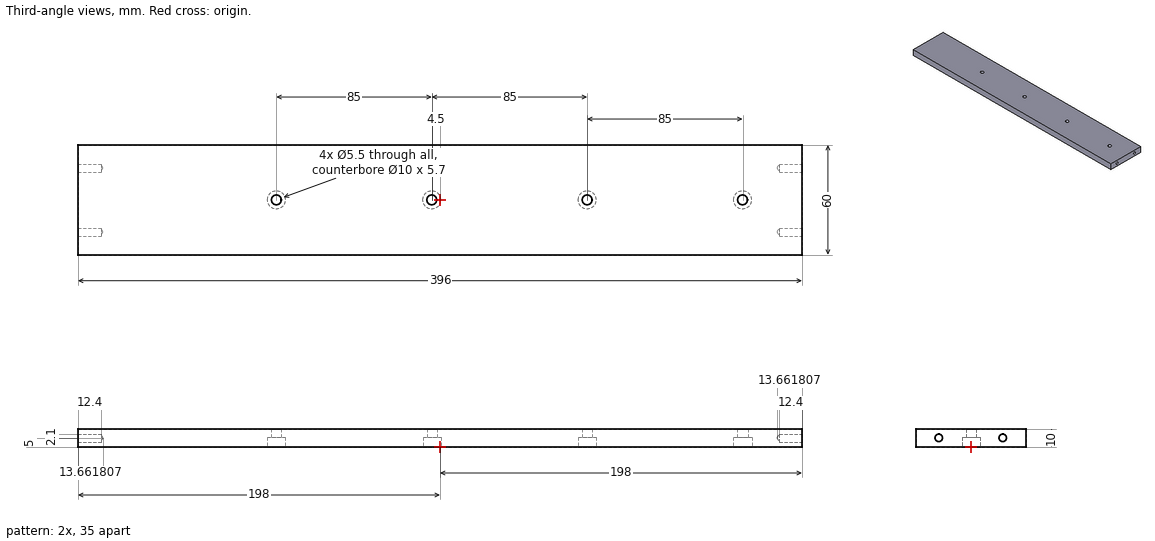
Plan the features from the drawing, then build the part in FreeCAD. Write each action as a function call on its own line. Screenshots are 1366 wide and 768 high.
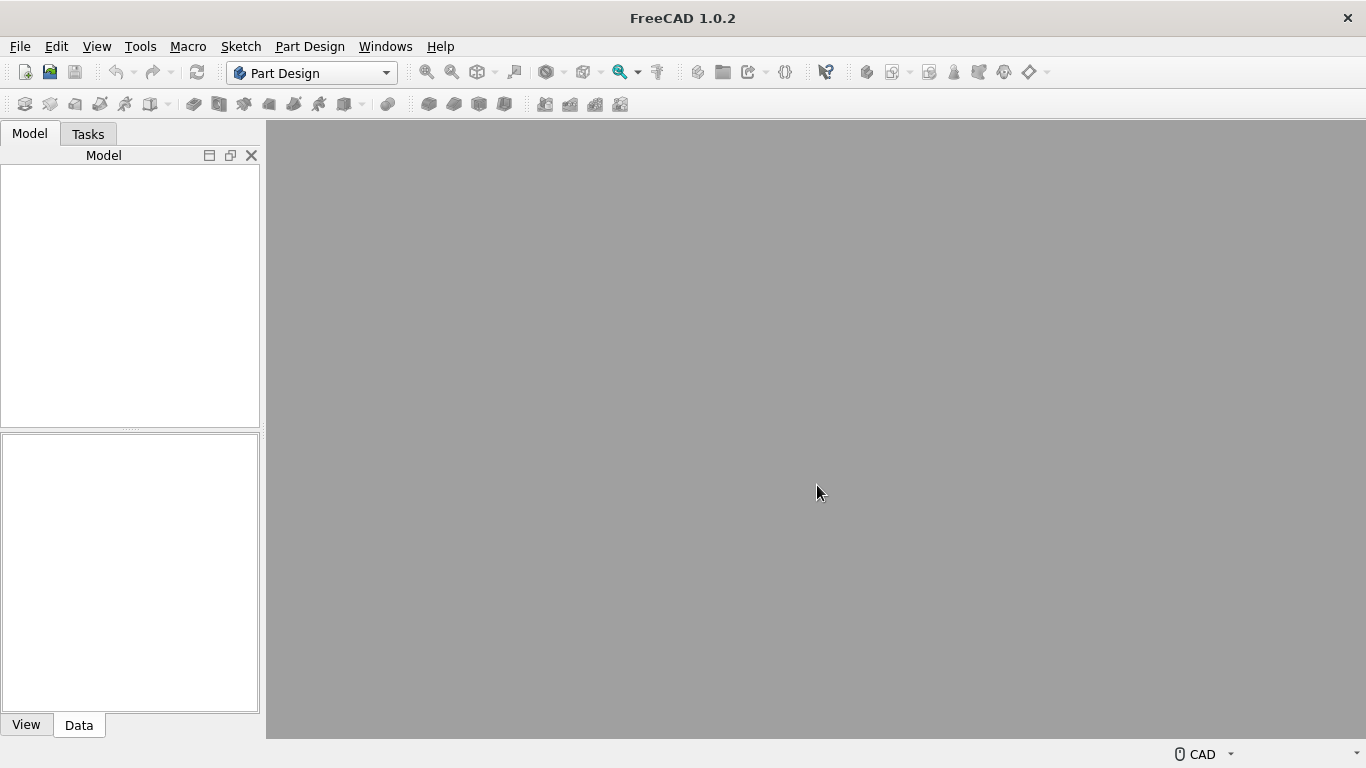
click(25, 72)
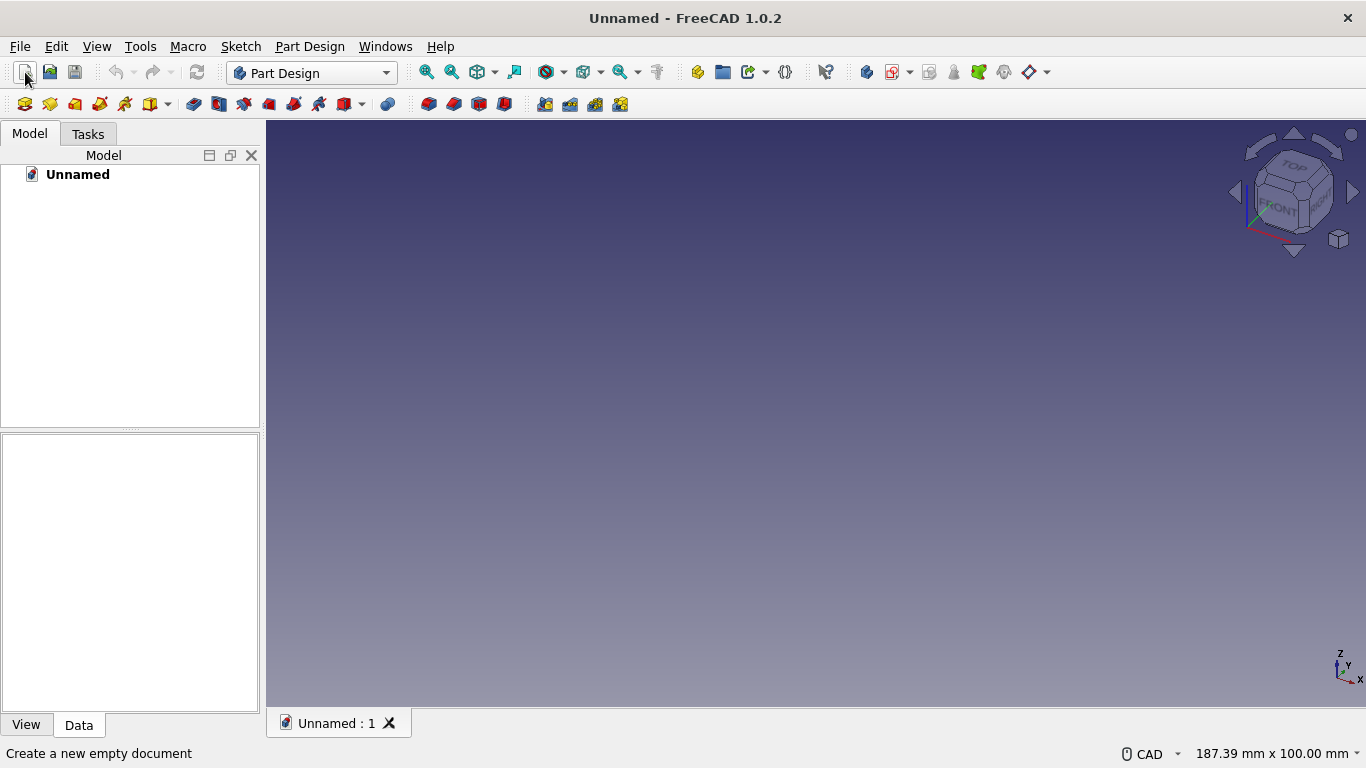
click(892, 72)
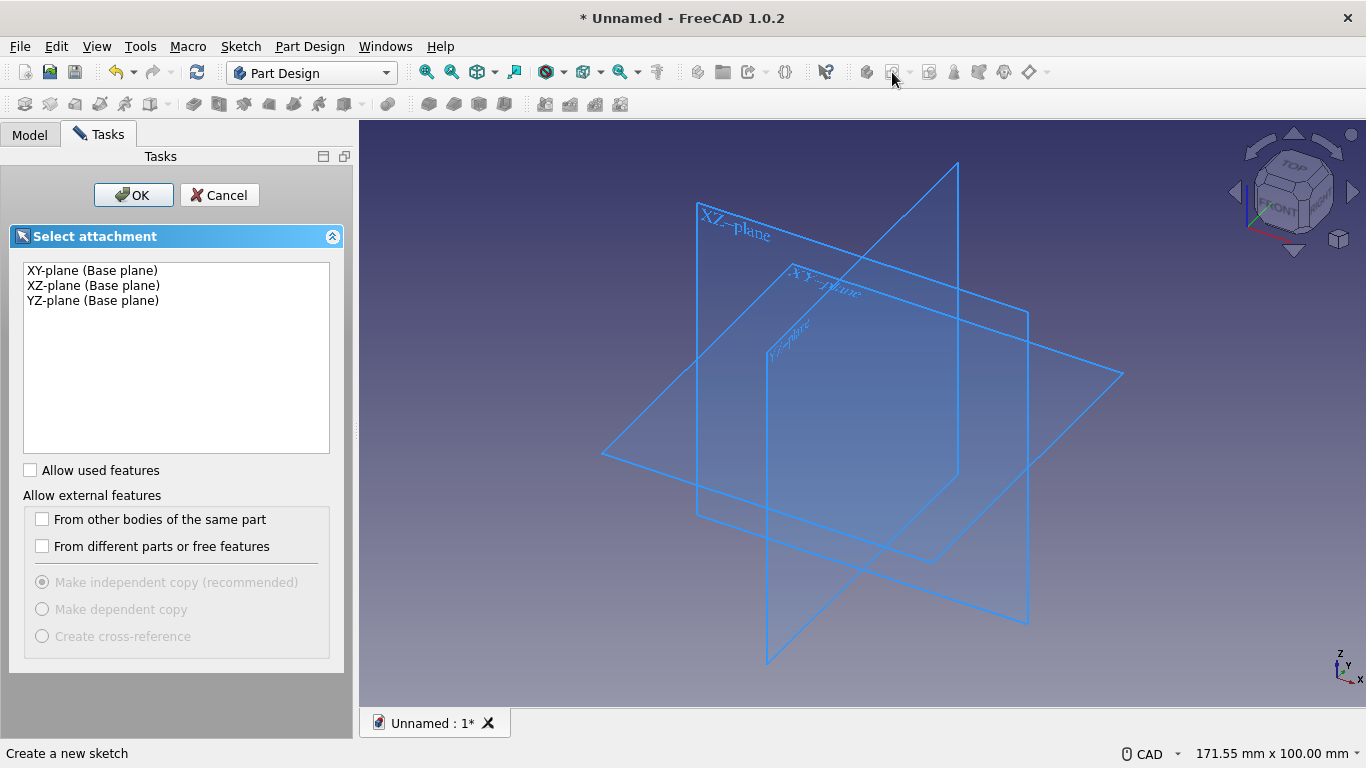
click(84, 270)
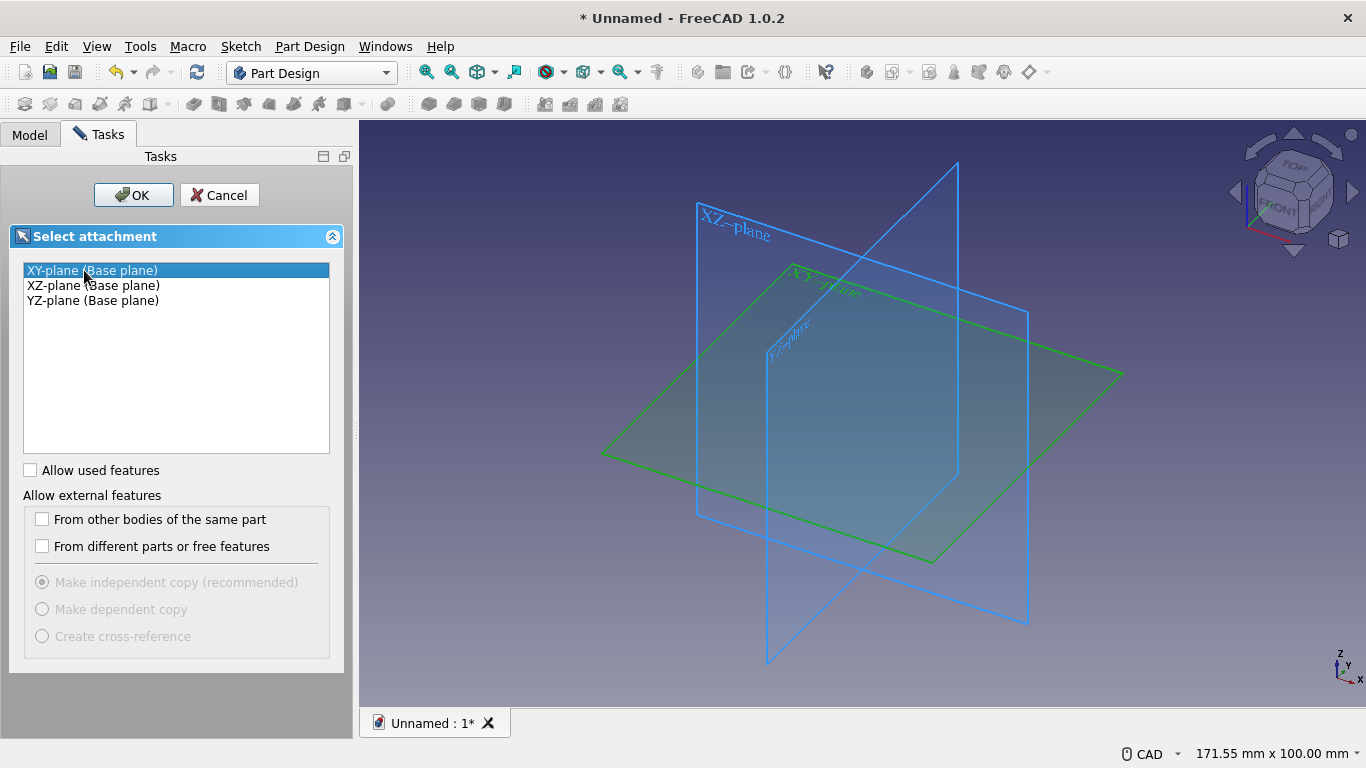
click(134, 195)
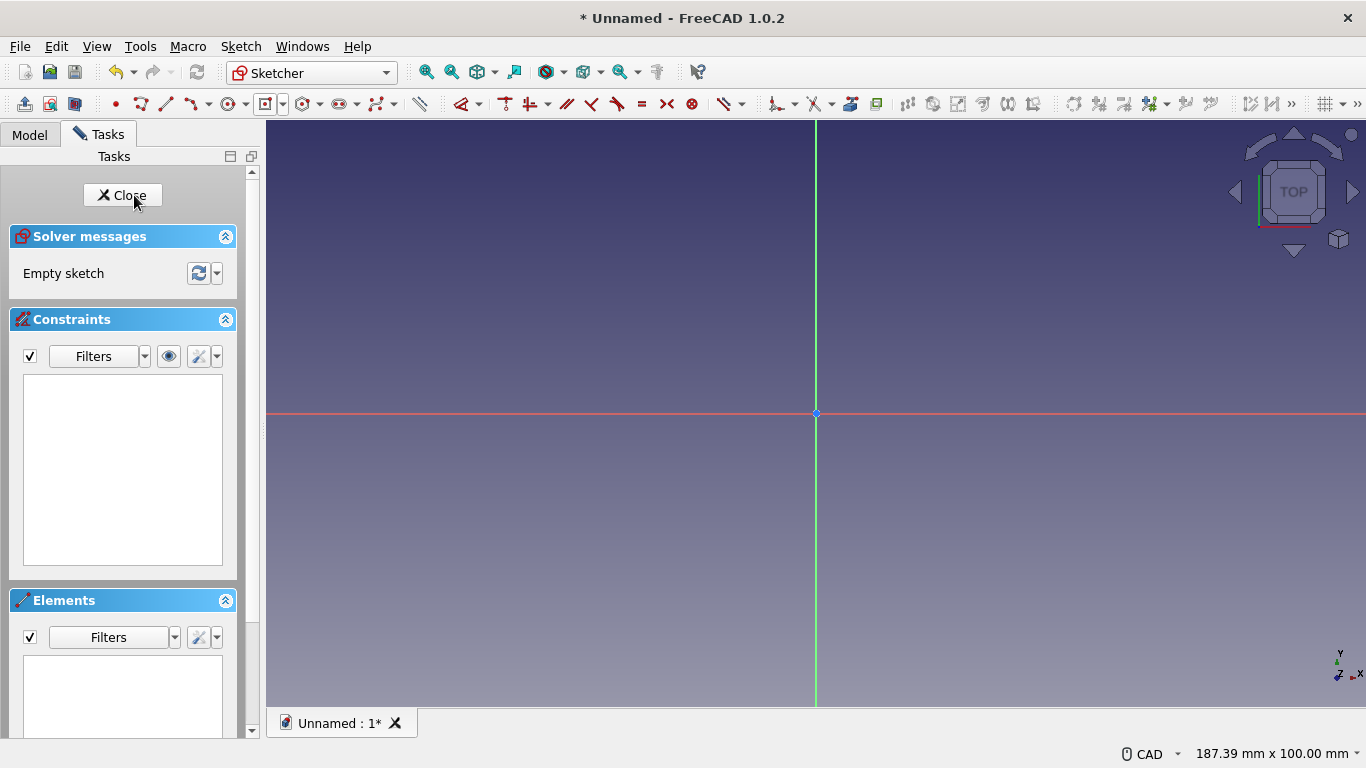
scroll(718, 413, down, 6)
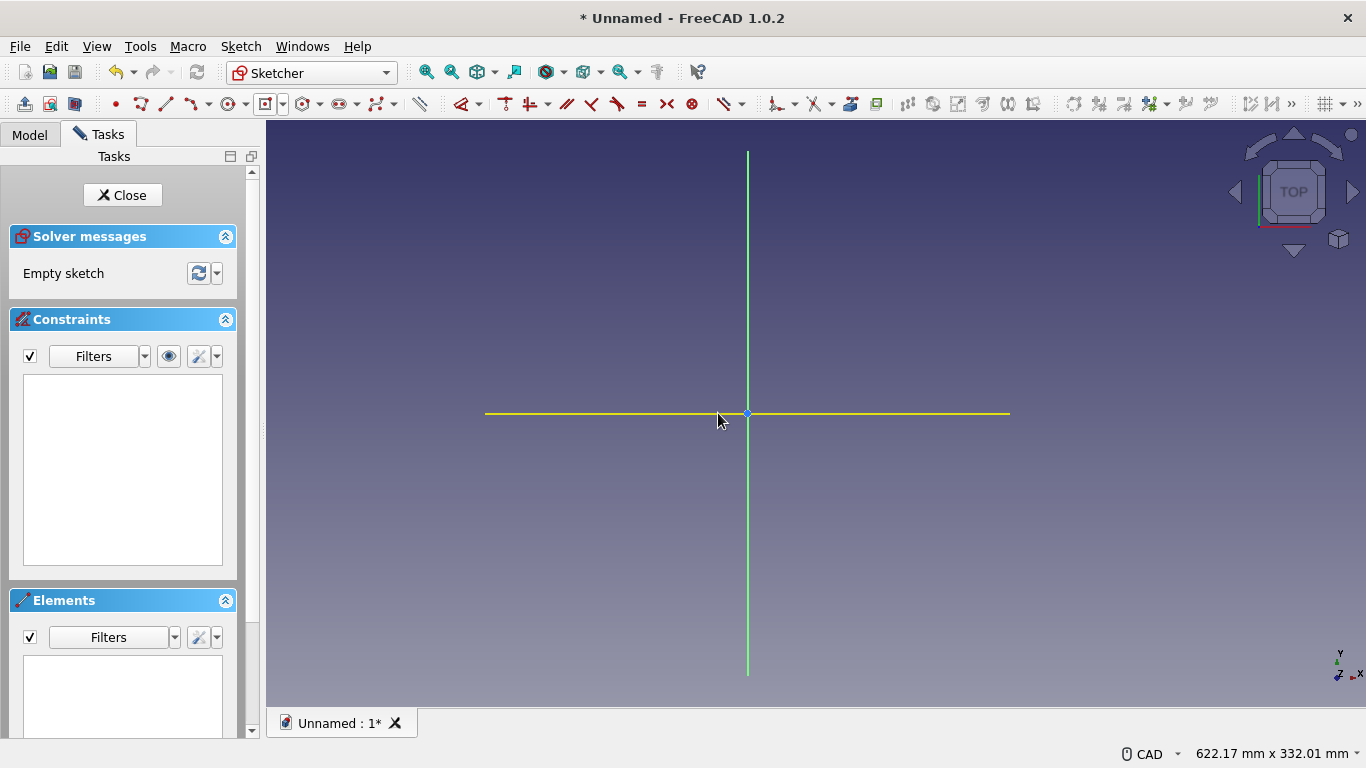
click(264, 104)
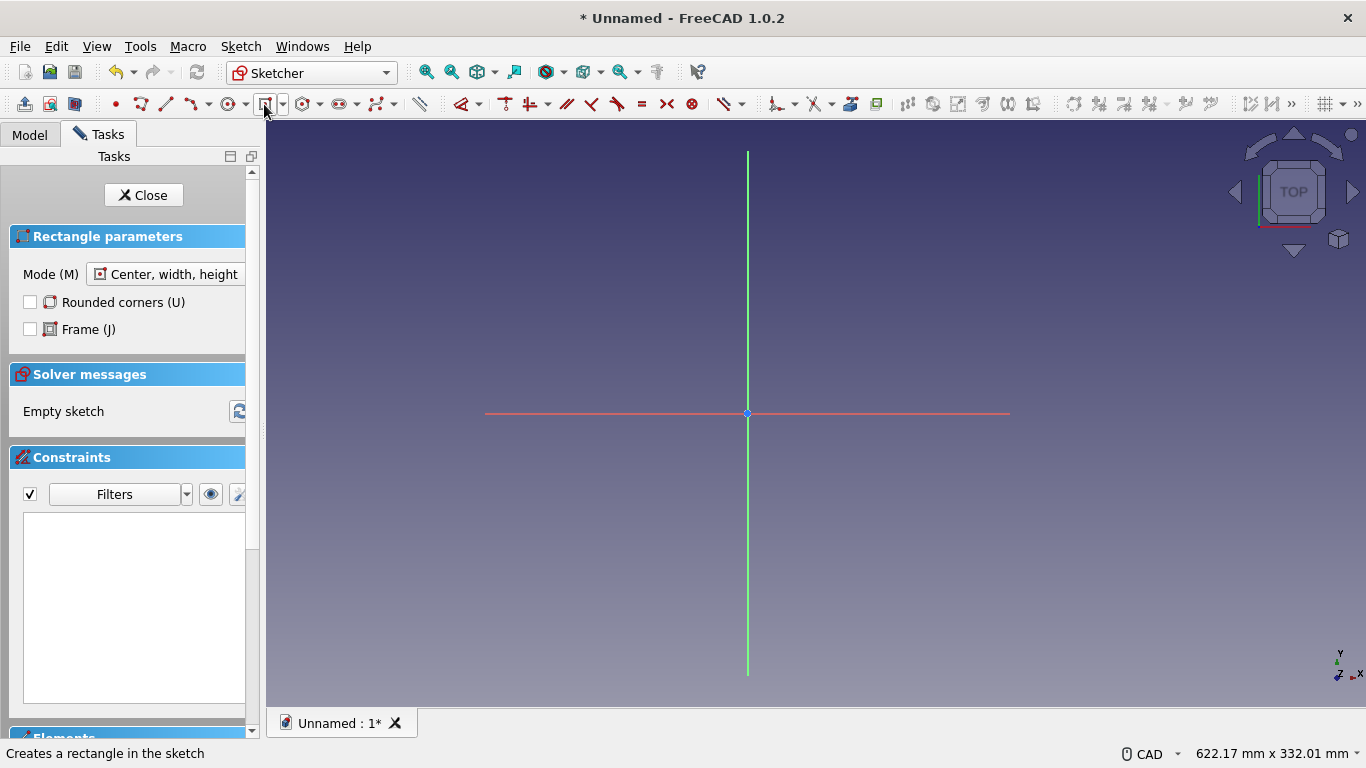
click(748, 414)
move(1098, 360)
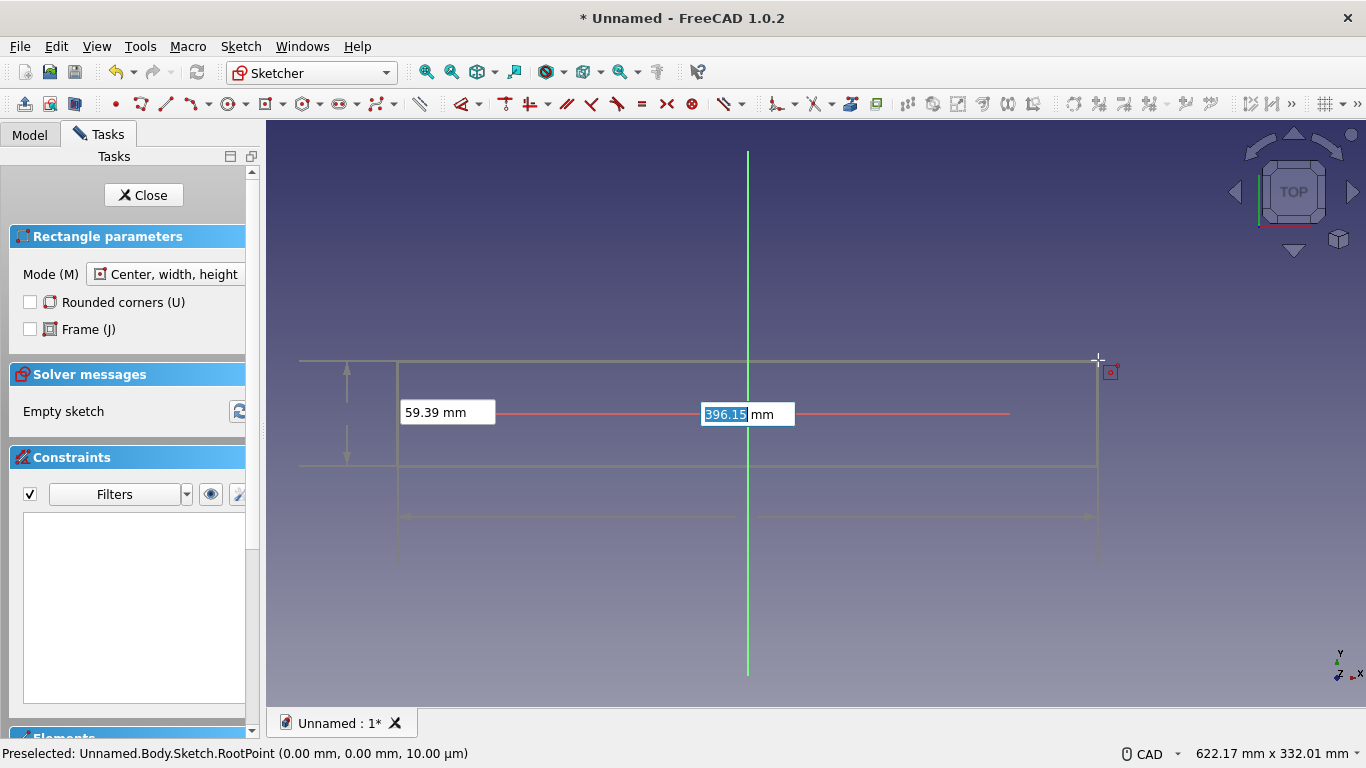
text(396)
key(Tab)
text(60)
key(Return)
key(Escape)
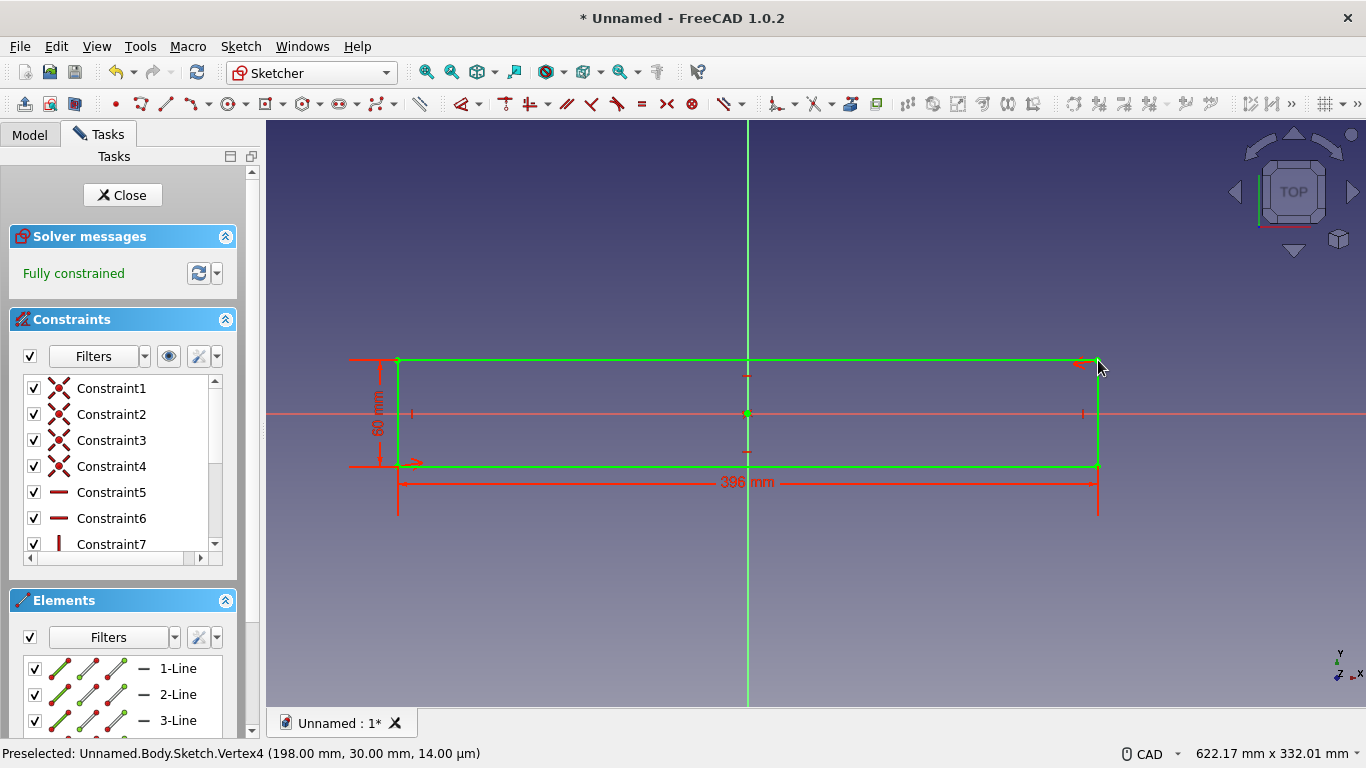
click(123, 195)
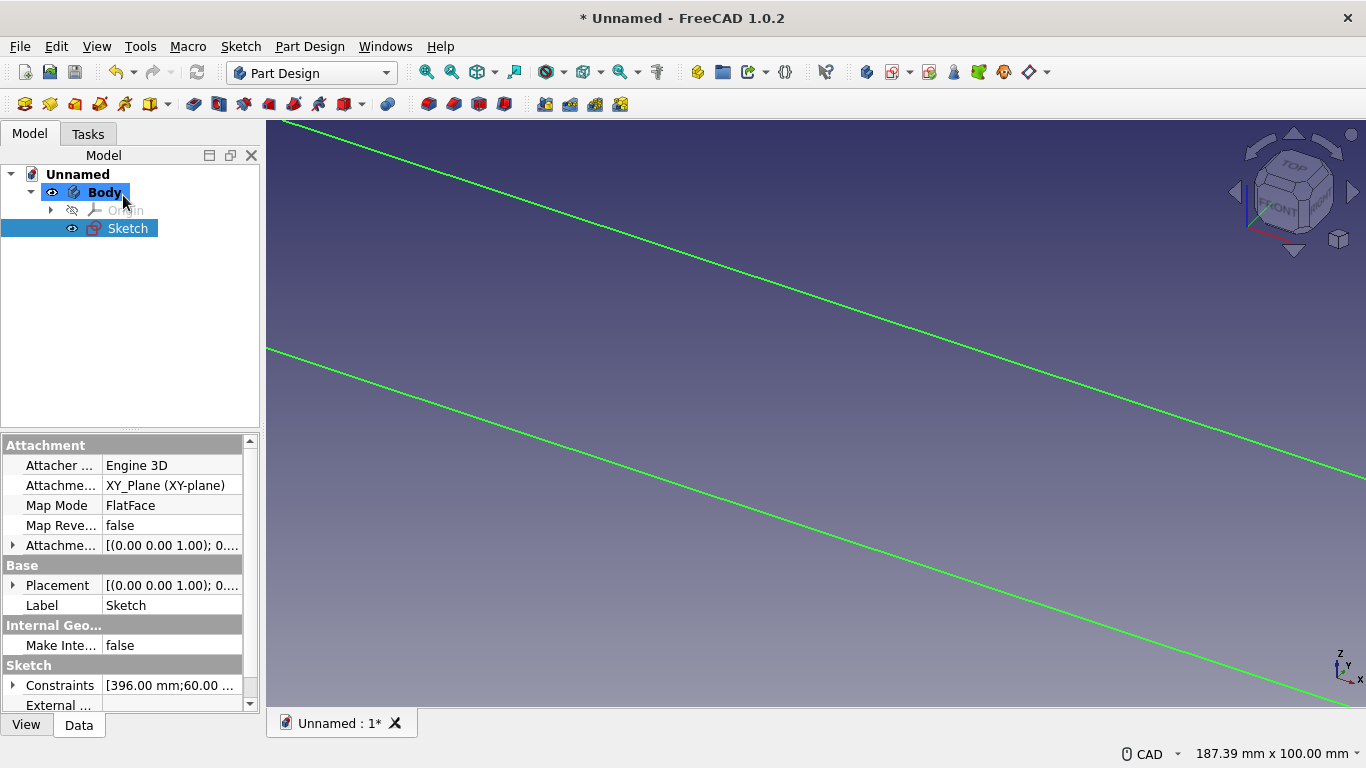
click(25, 104)